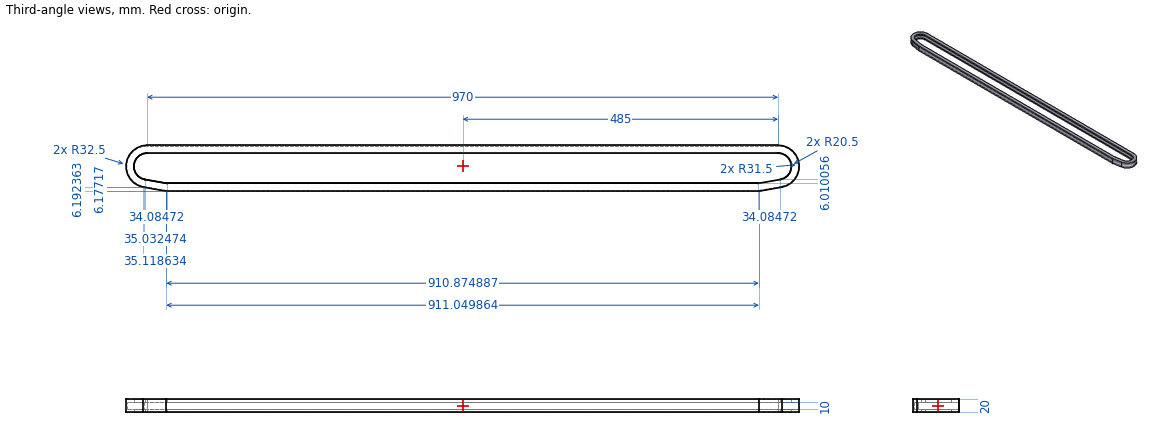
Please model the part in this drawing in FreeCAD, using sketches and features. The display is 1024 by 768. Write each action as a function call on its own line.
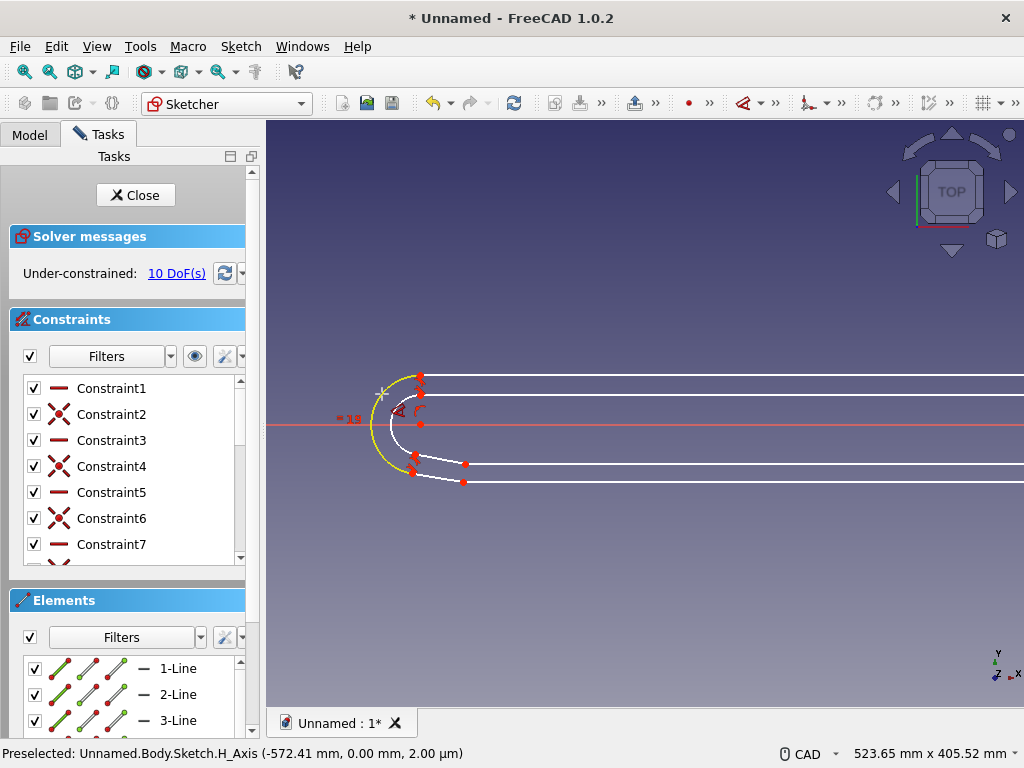
click(382, 394)
click(357, 374)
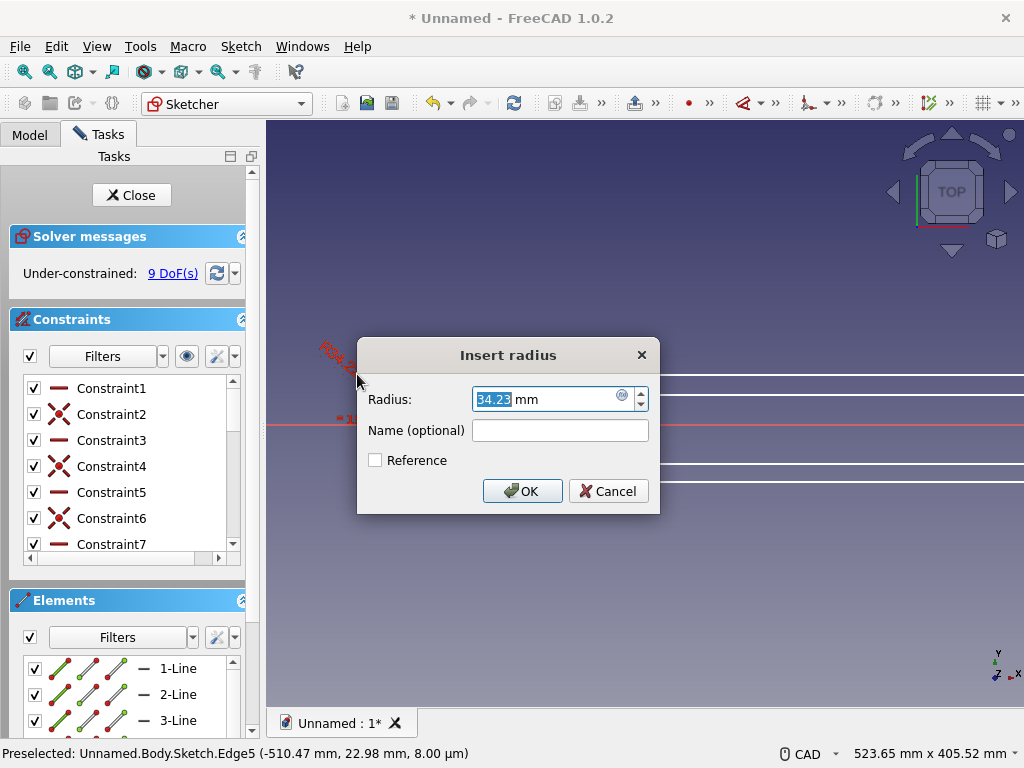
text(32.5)
key(Return)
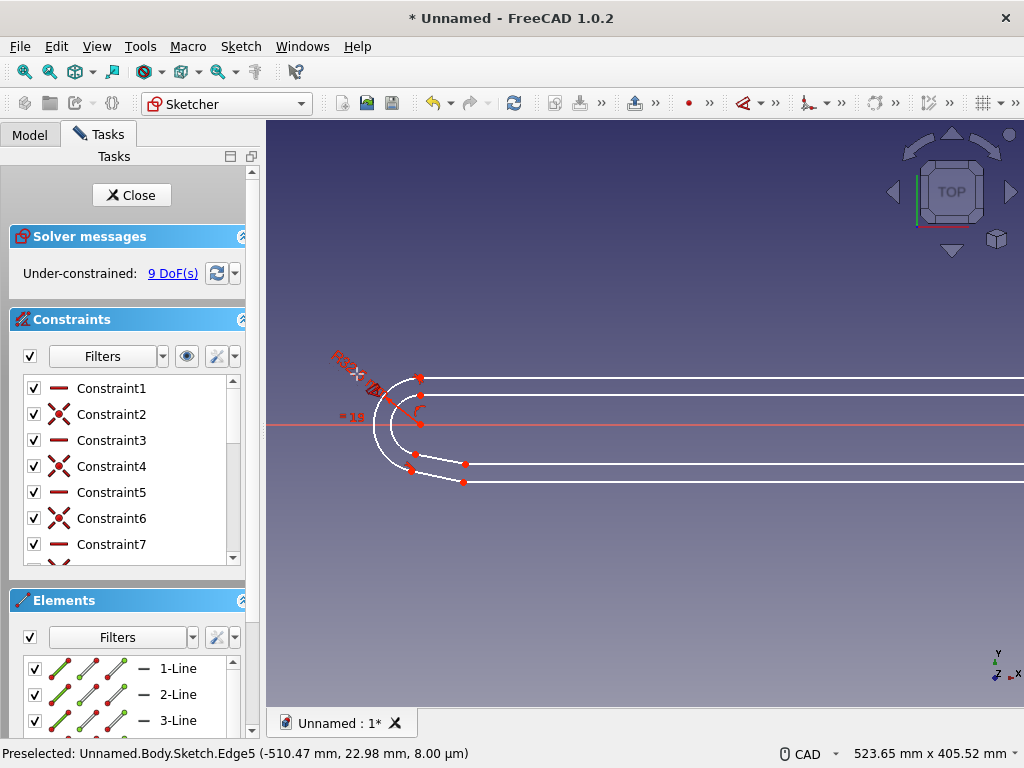
scroll(398, 408, down, 7)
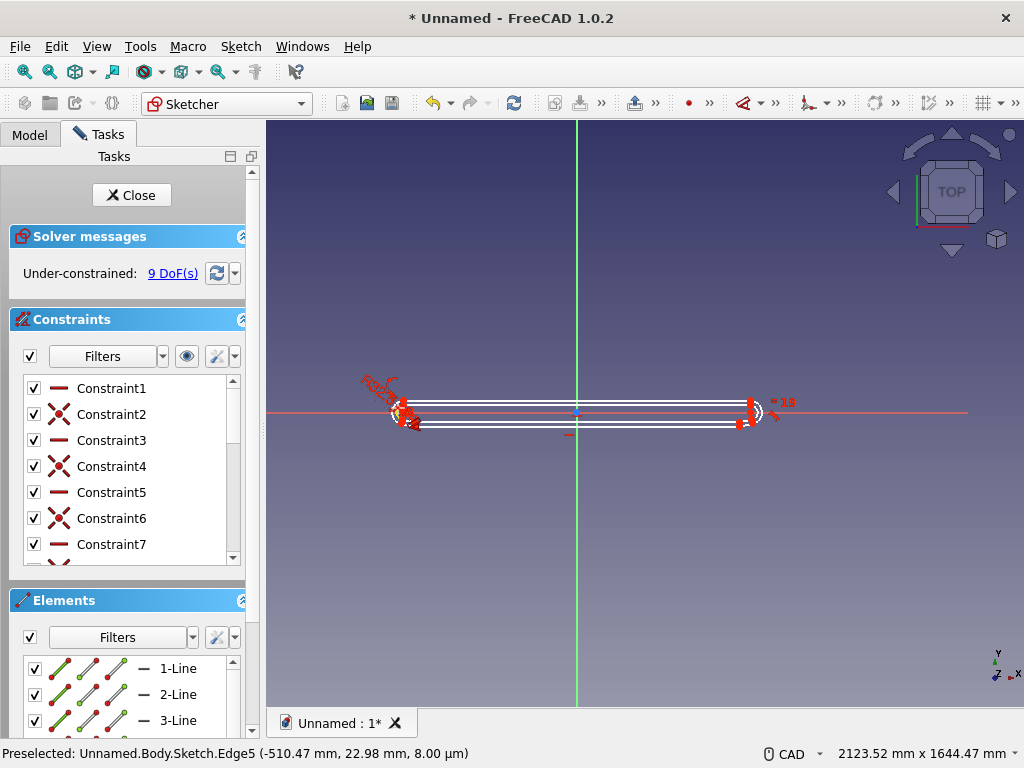
scroll(757, 416, up, 9)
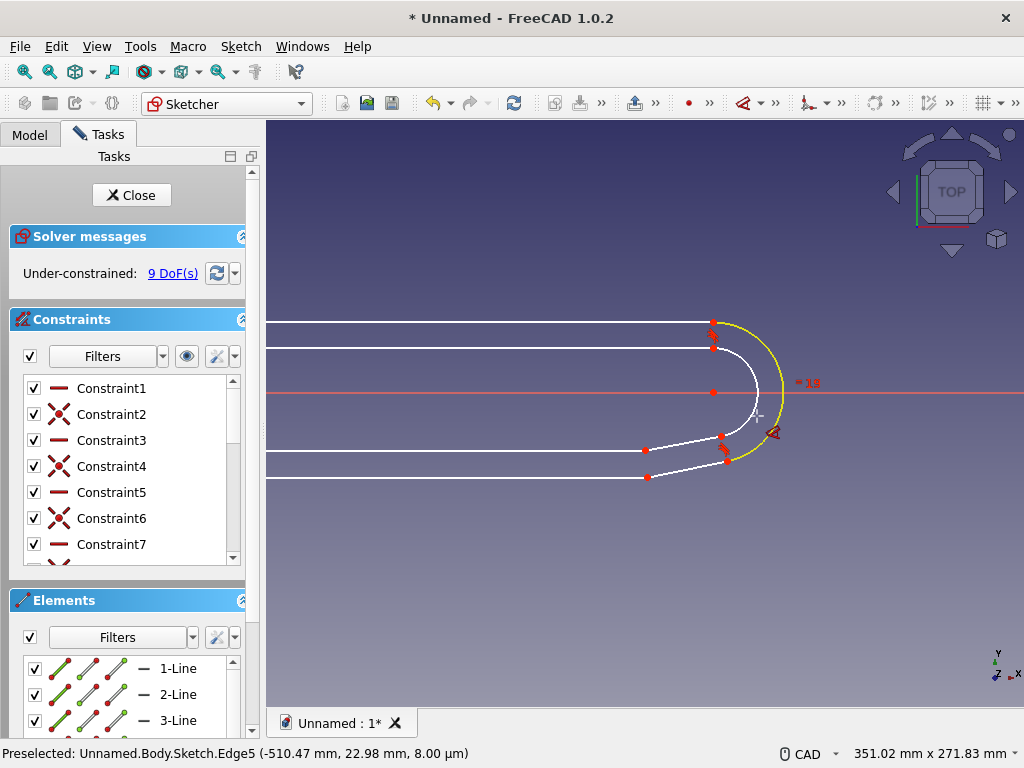
click(752, 414)
click(800, 441)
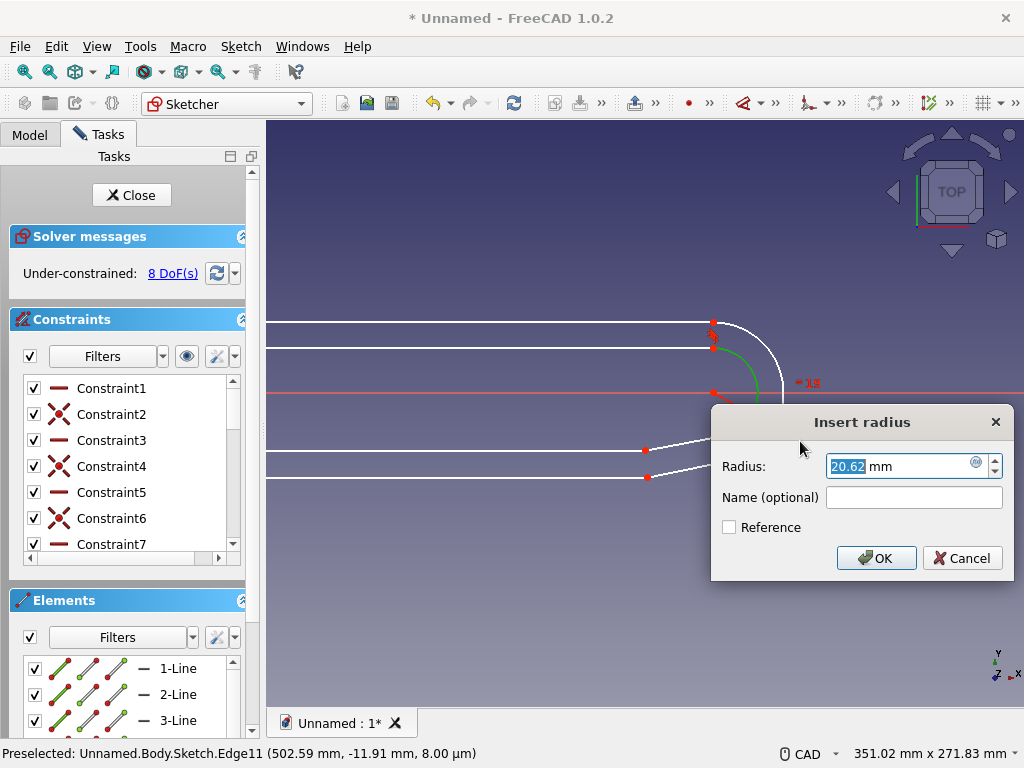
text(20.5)
key(Return)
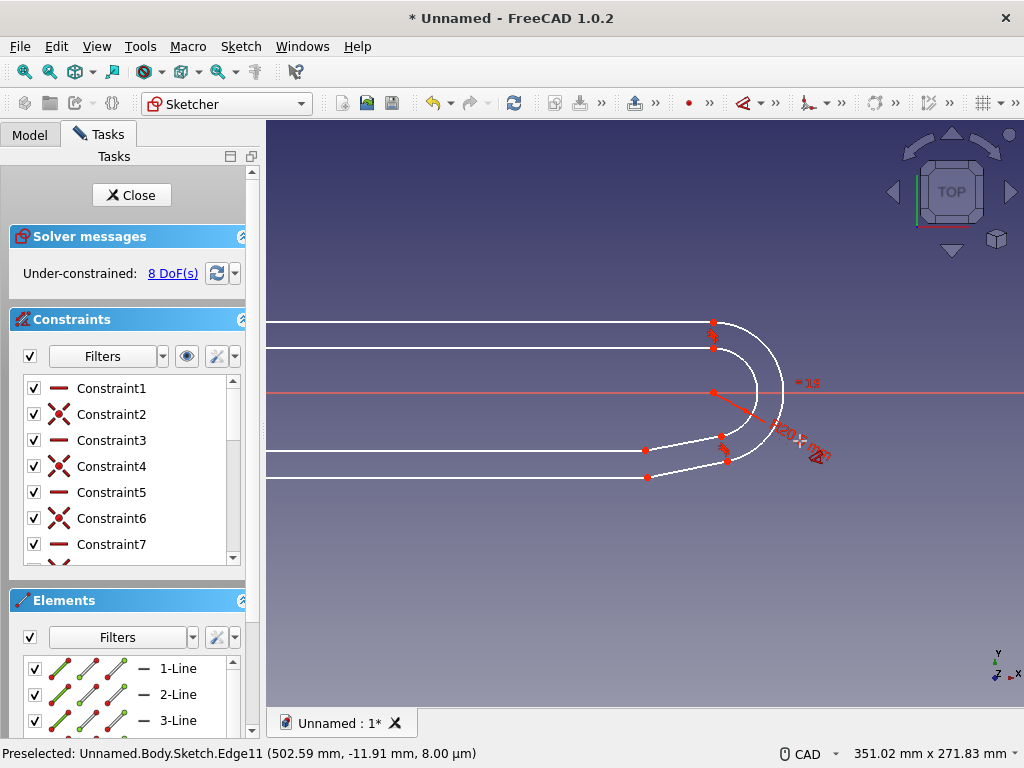
scroll(757, 416, down, 9)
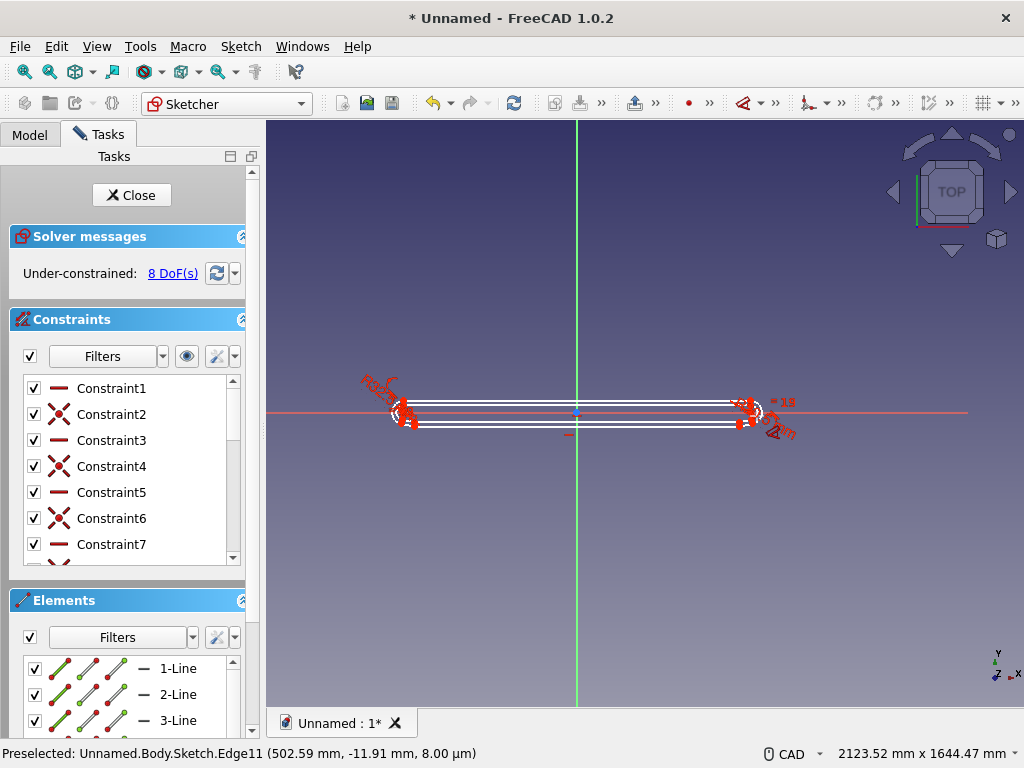
scroll(646, 401, up, 6)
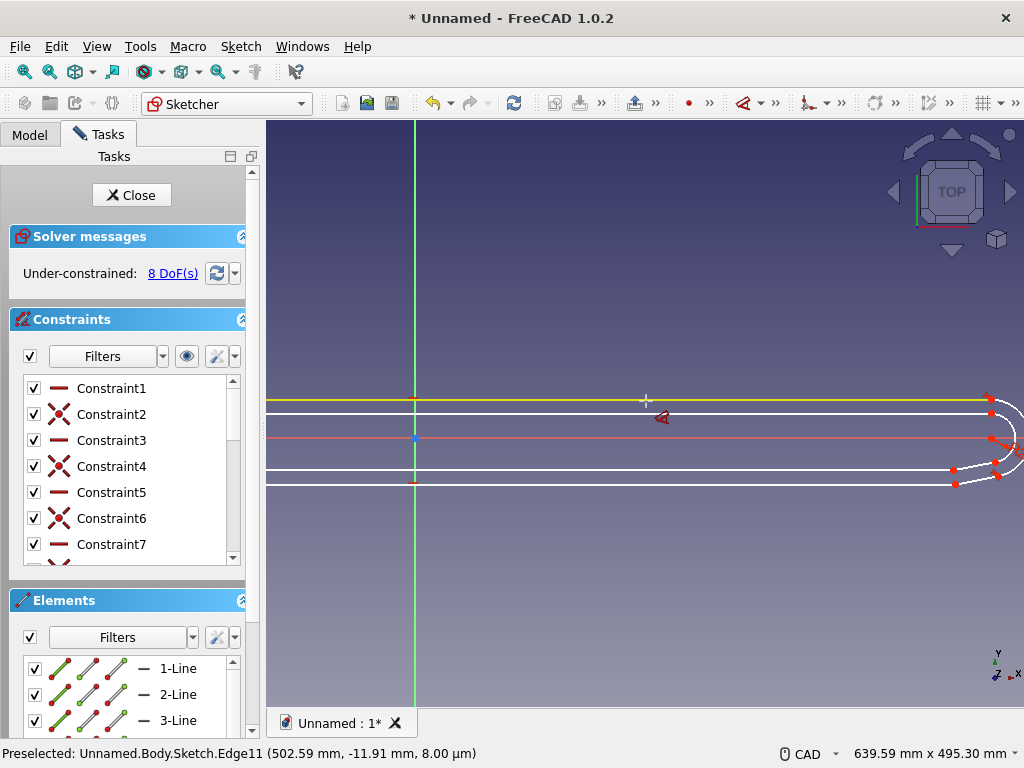
click(646, 400)
click(576, 366)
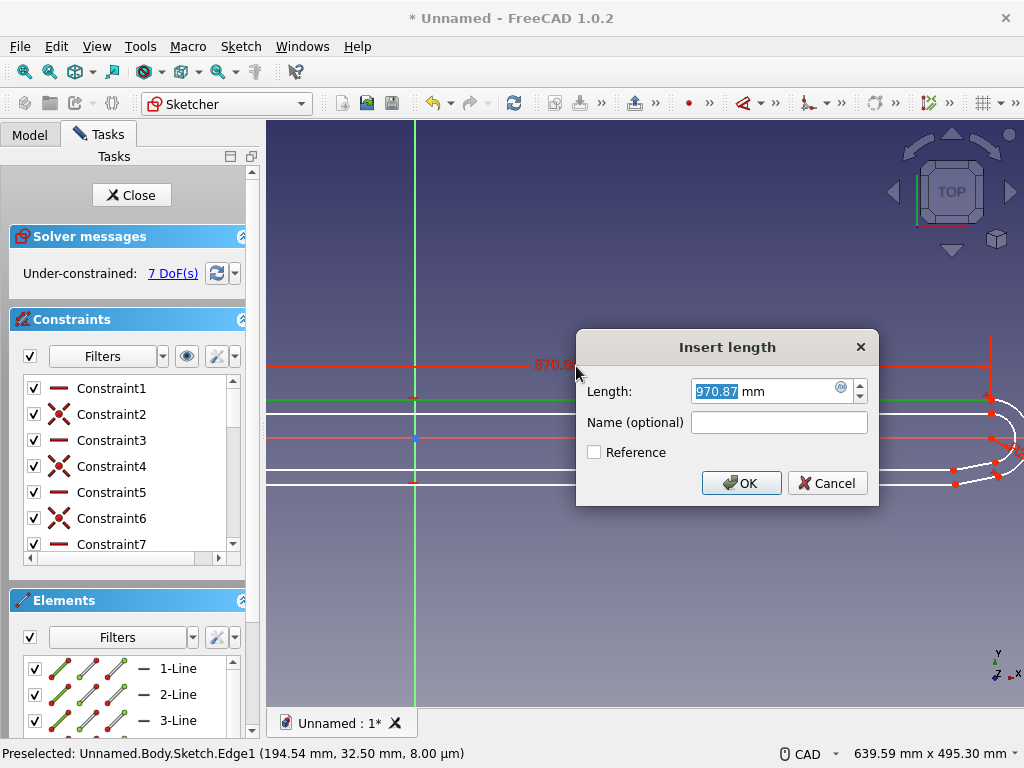
text(970)
key(Return)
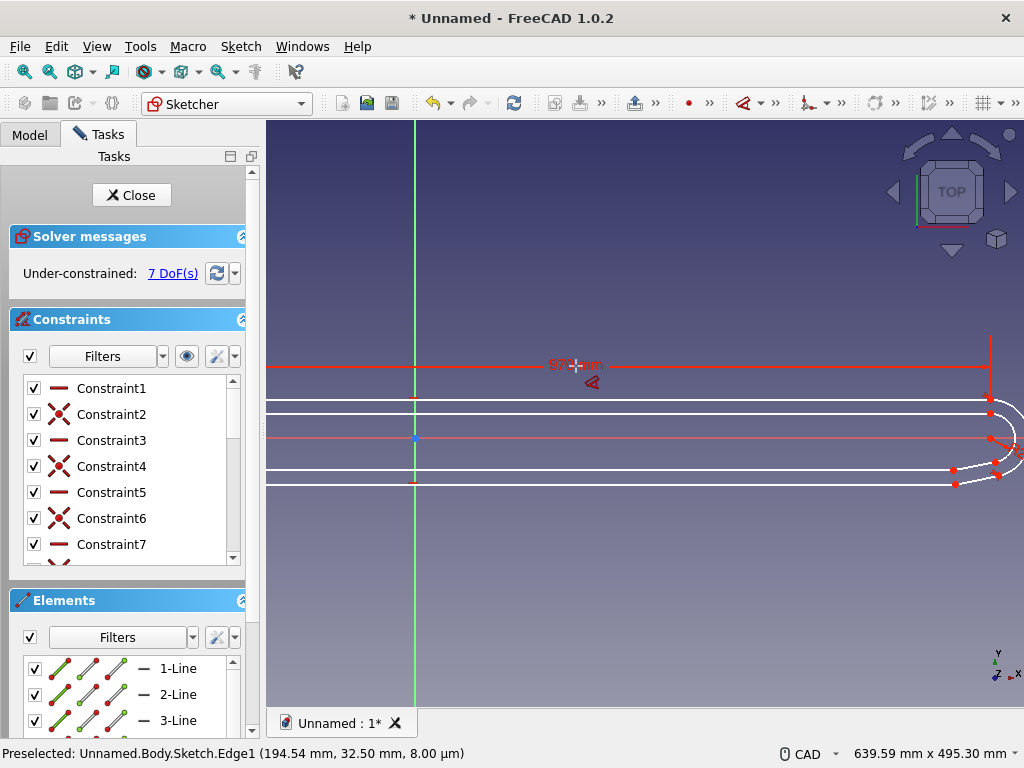
scroll(646, 401, down, 6)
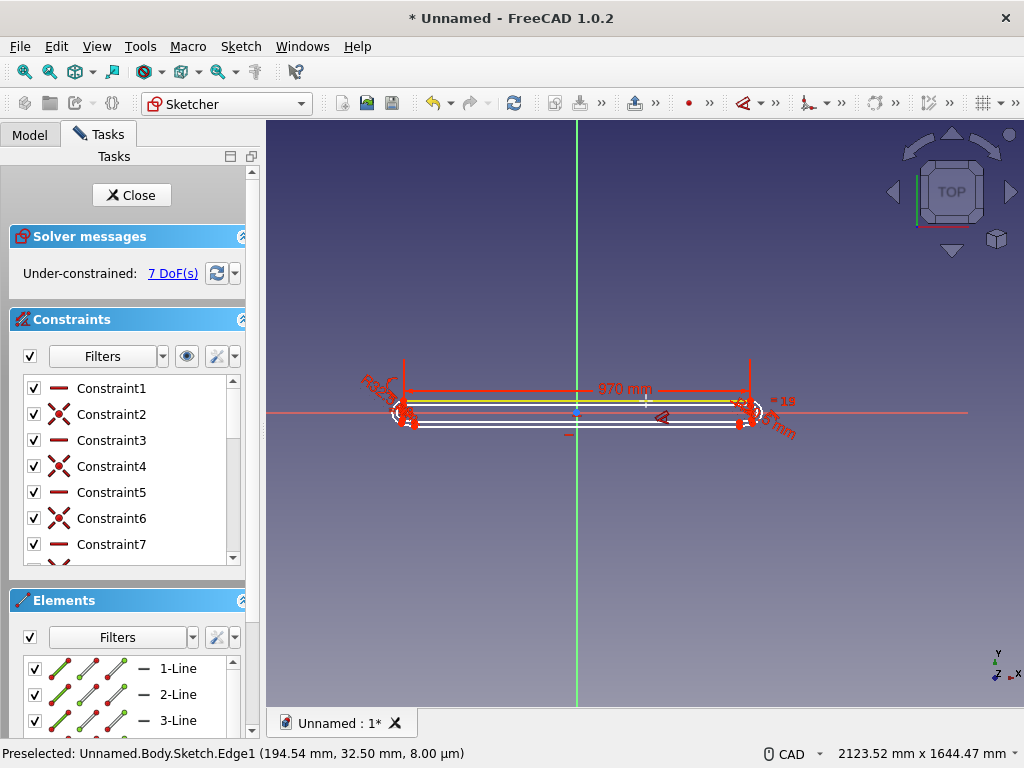
scroll(750, 401, up, 6)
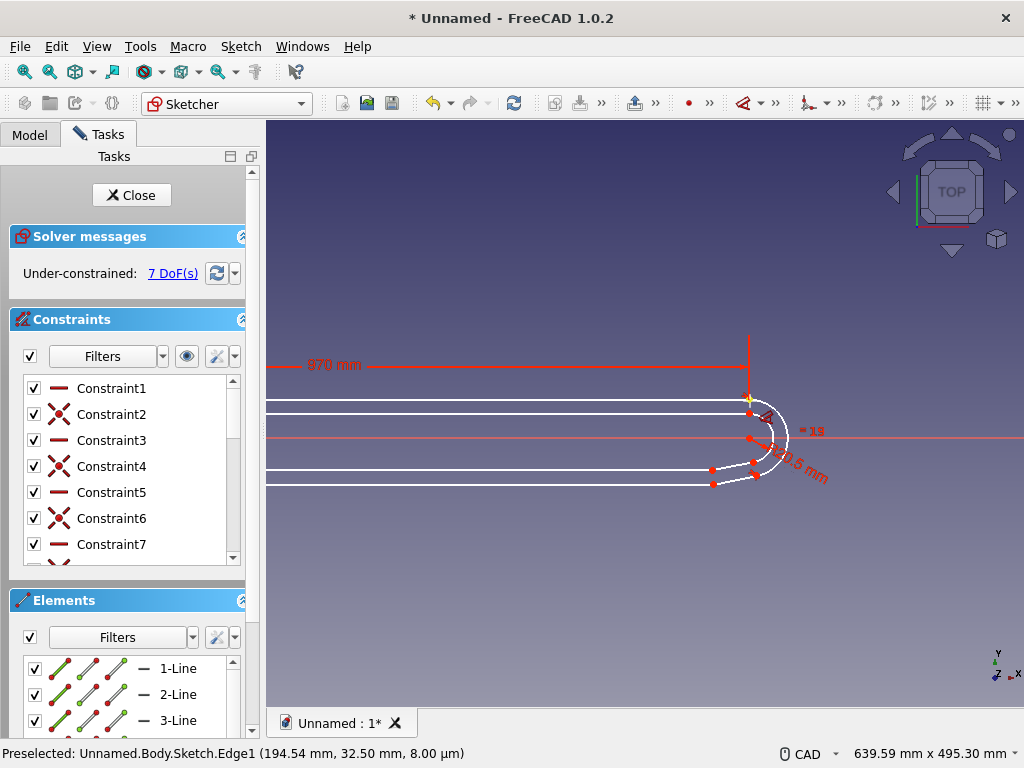
click(749, 400)
click(522, 366)